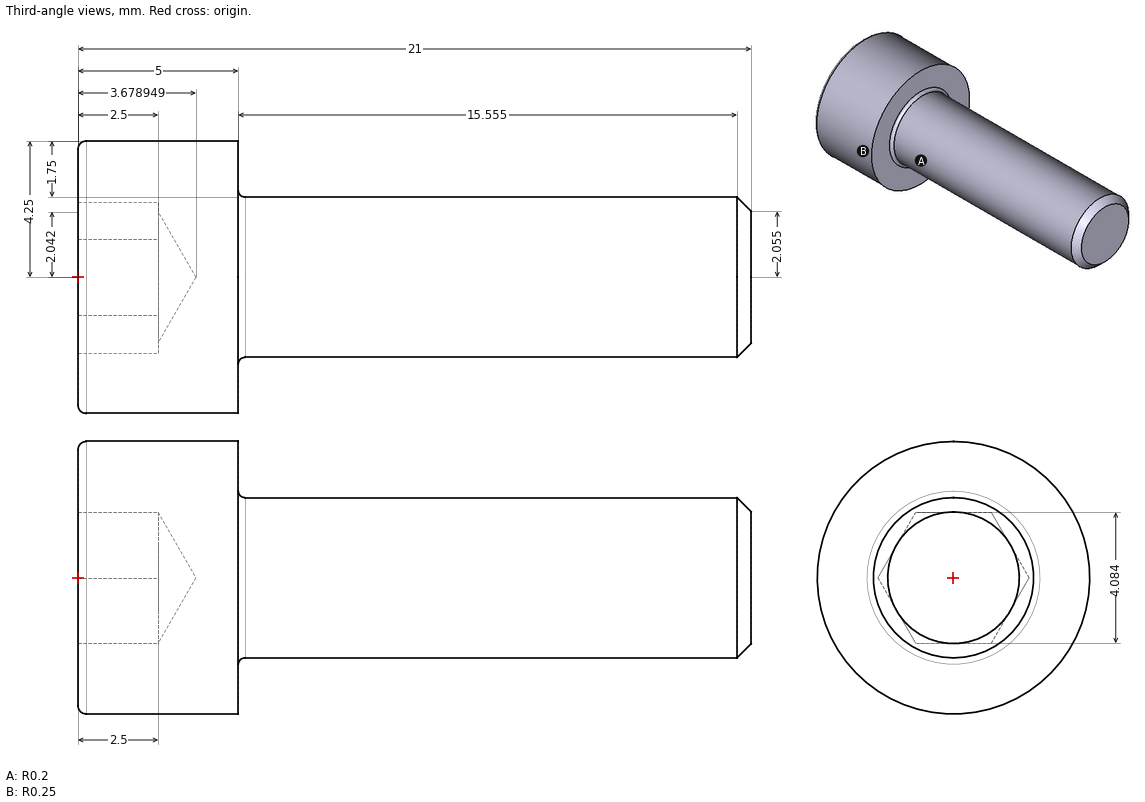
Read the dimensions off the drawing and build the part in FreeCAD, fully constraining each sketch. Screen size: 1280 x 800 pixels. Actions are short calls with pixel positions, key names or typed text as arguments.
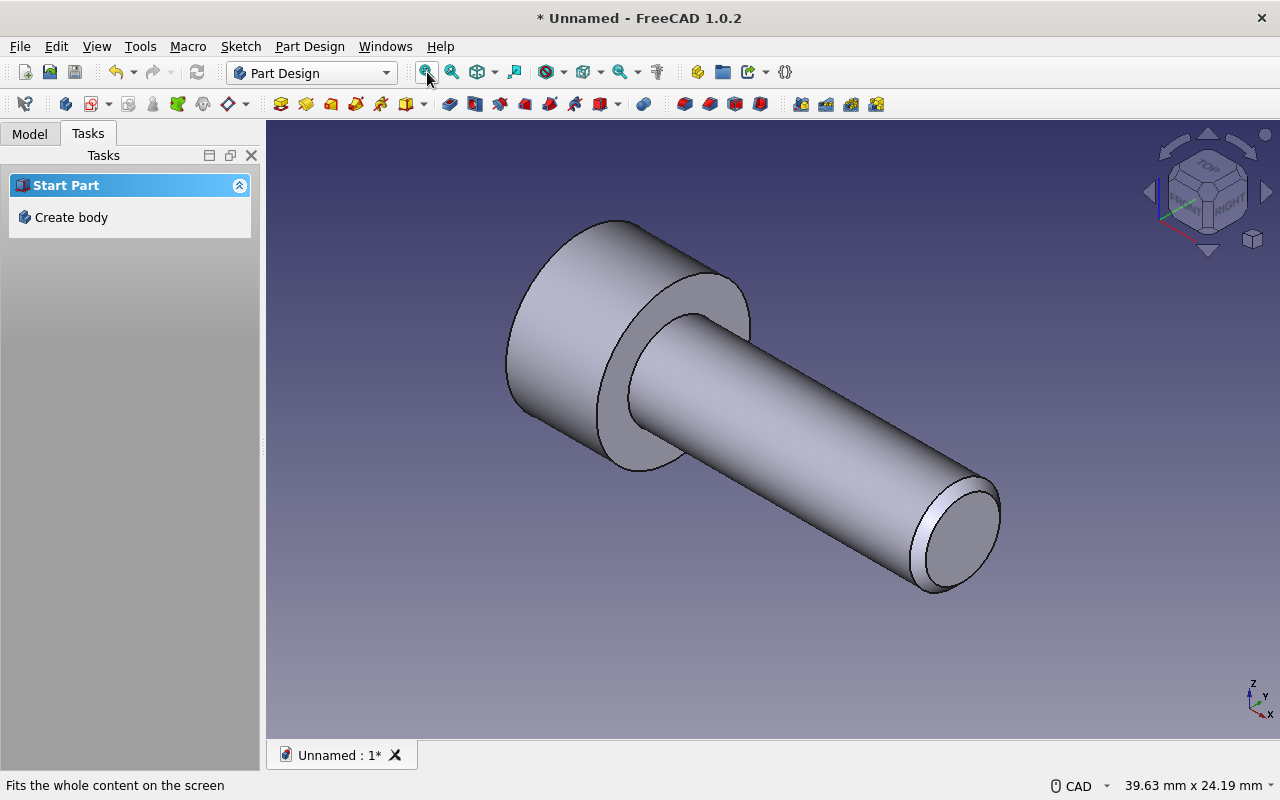
key(2)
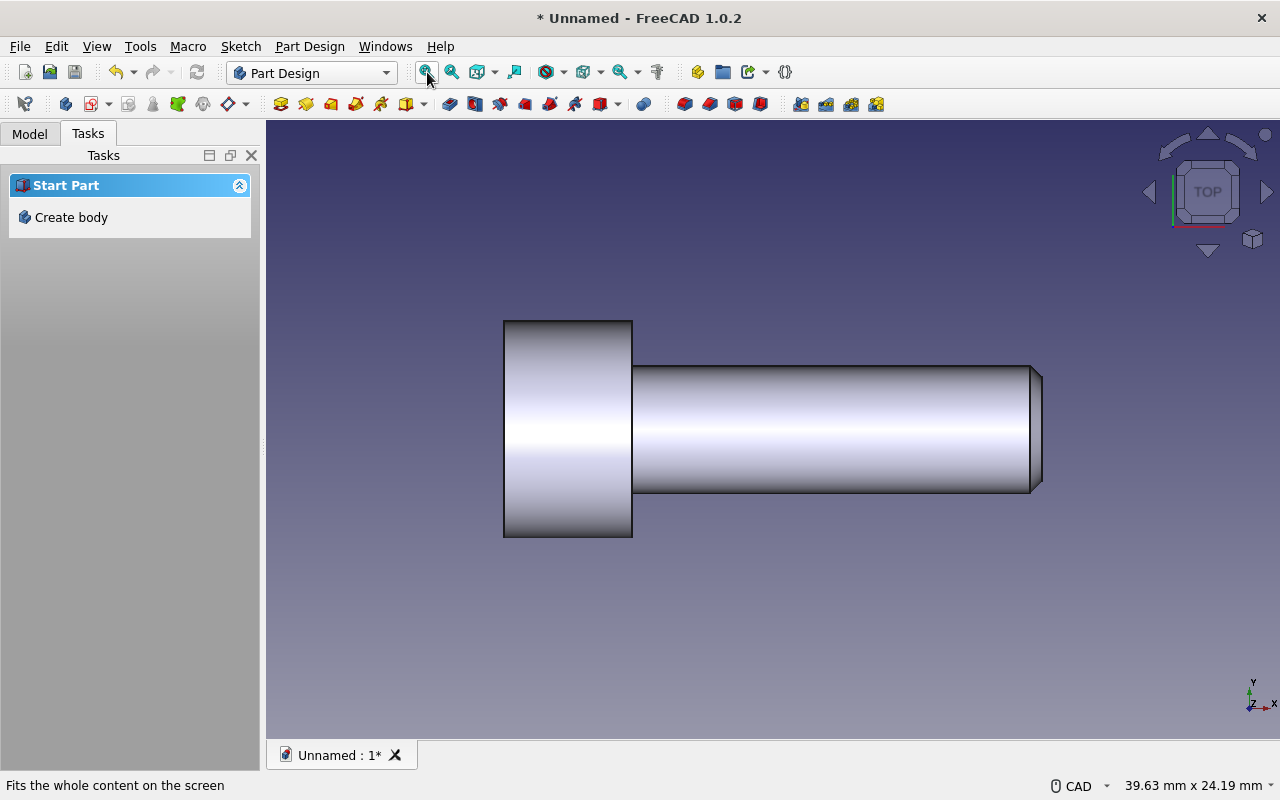
key(1)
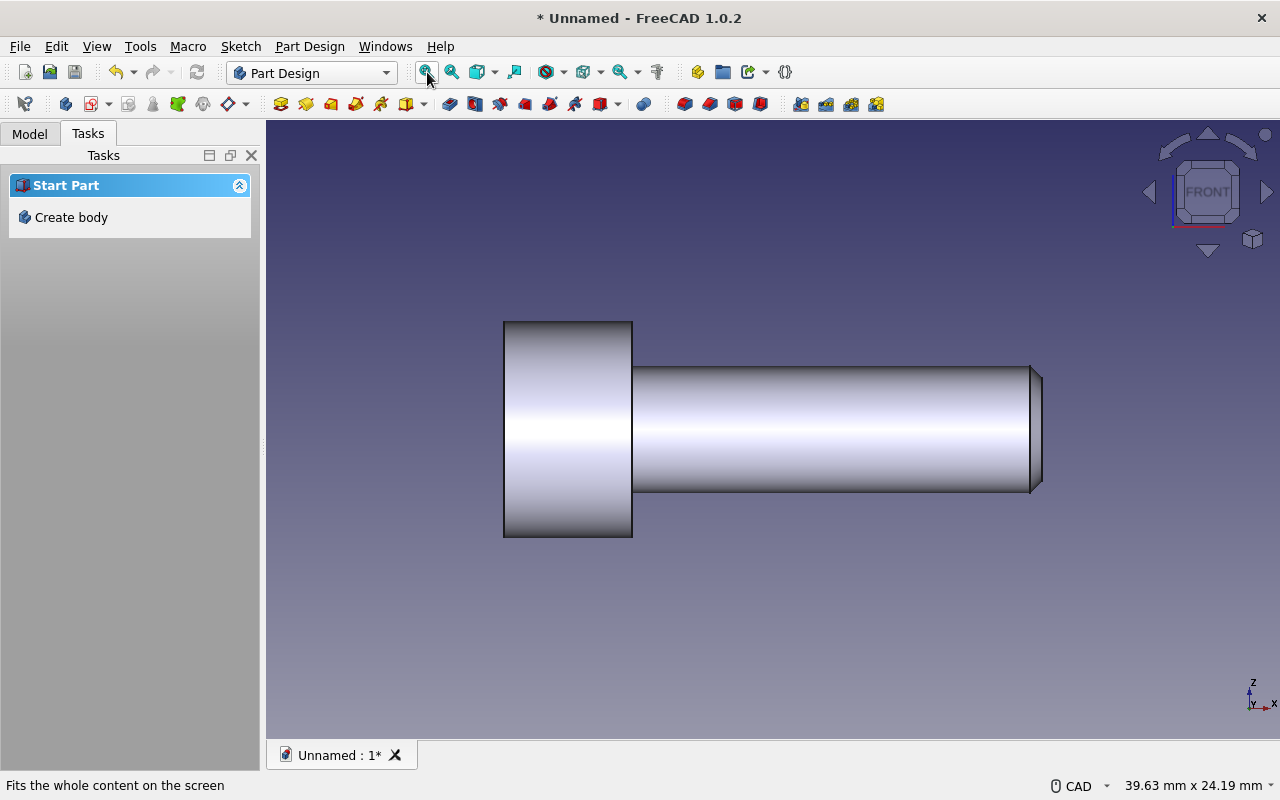
key(3)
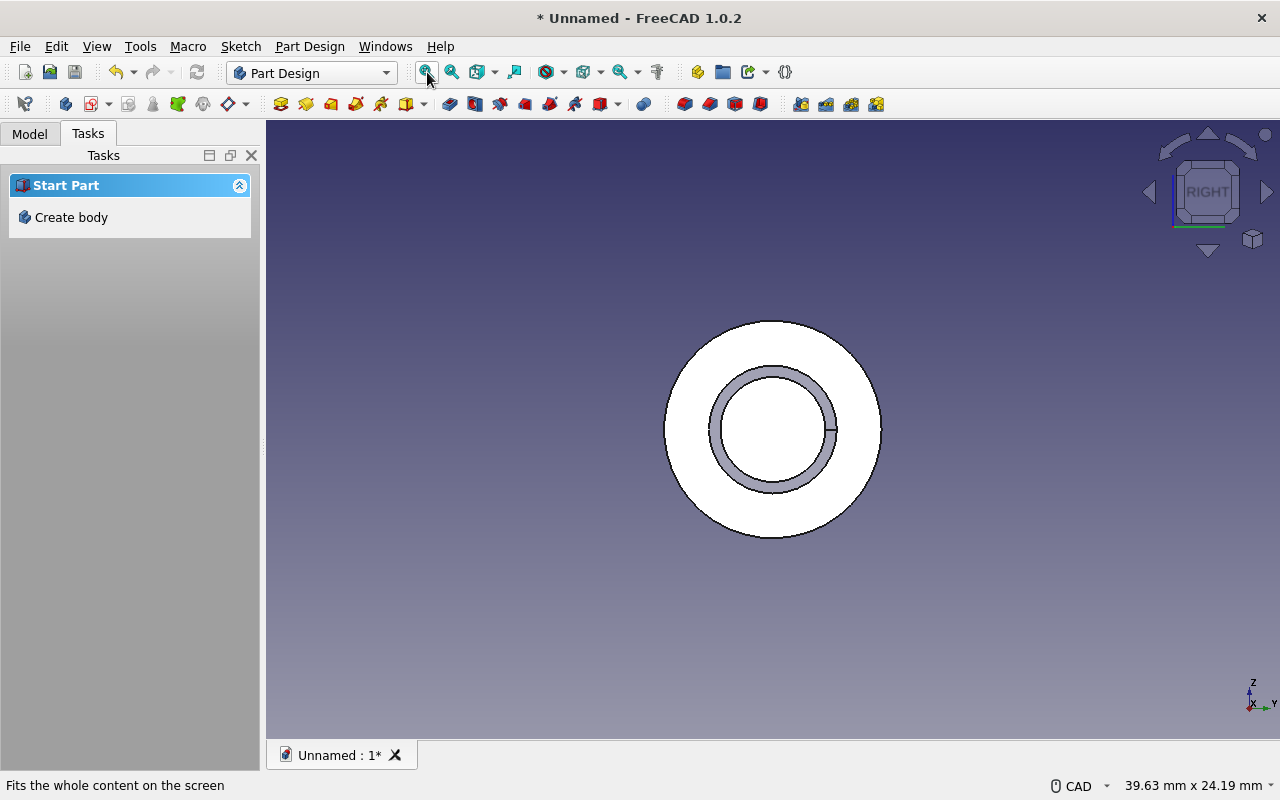
click(427, 72)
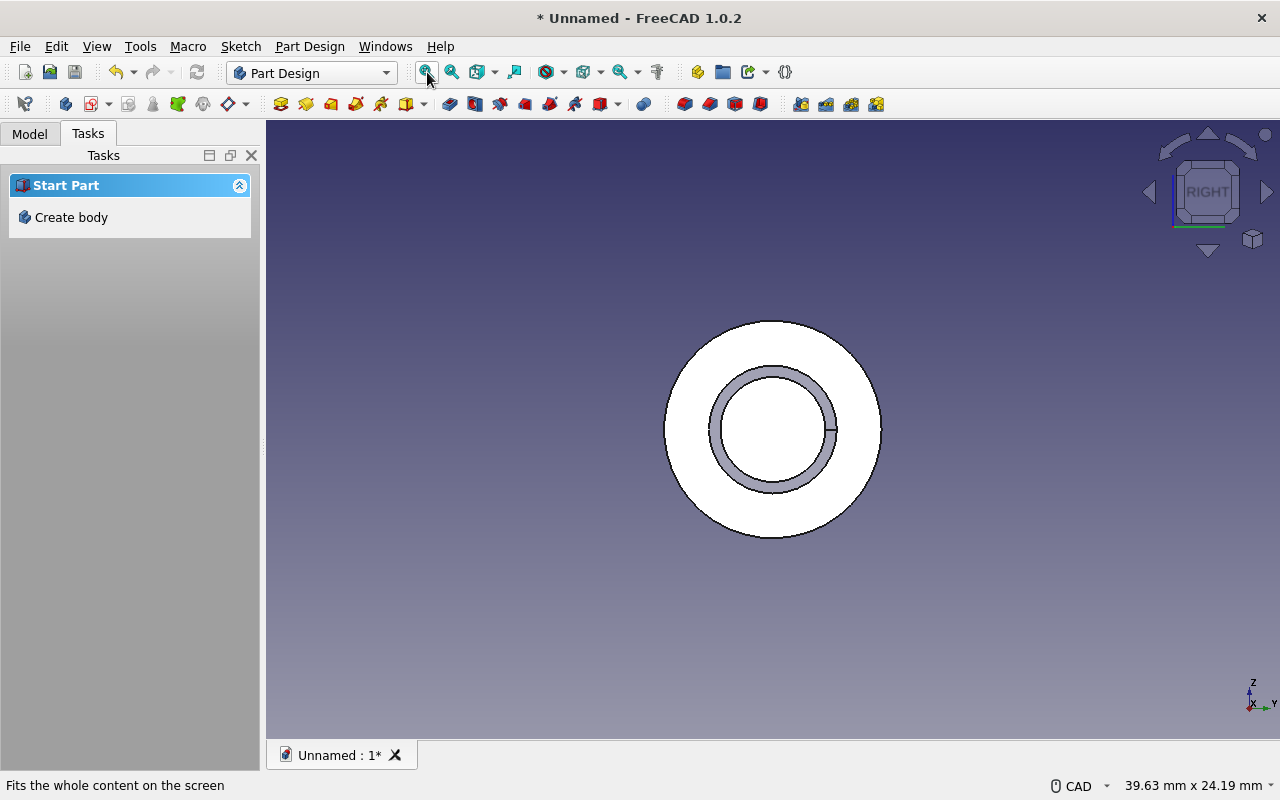
key(5)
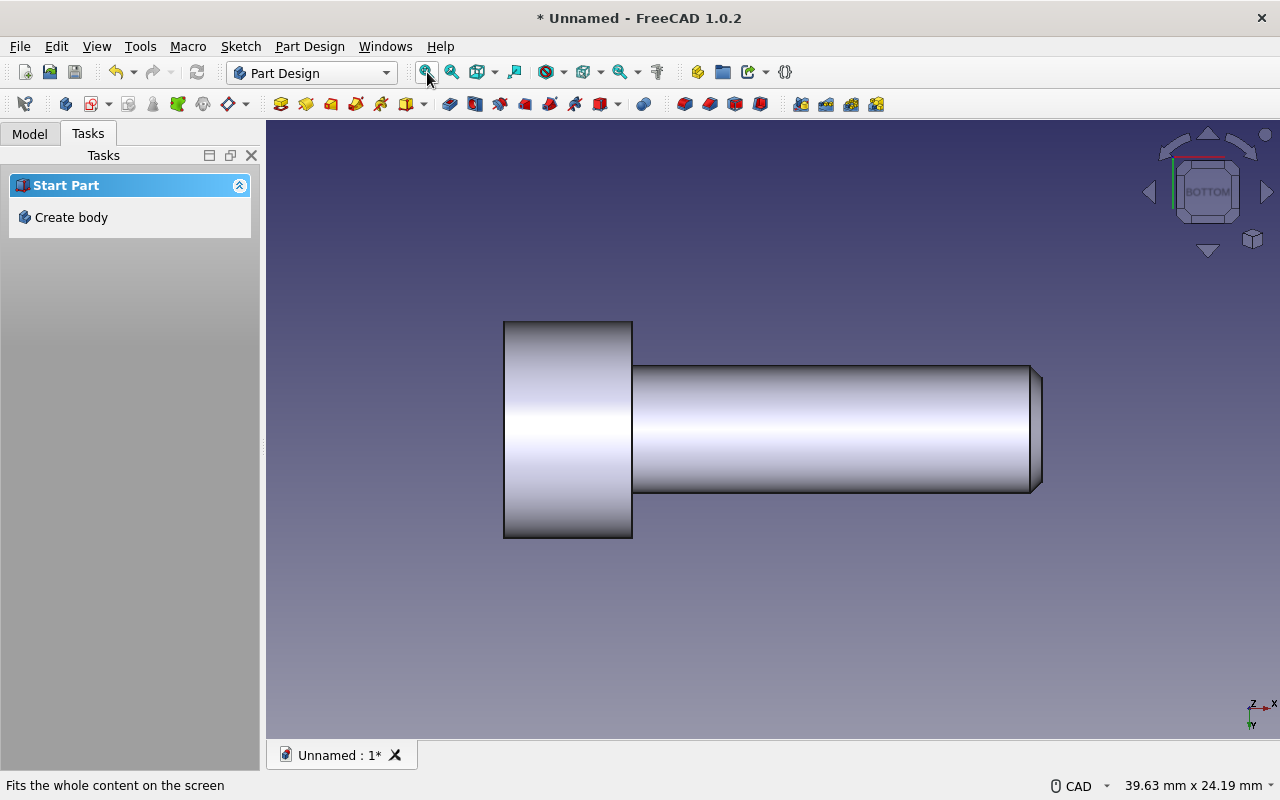
key(4)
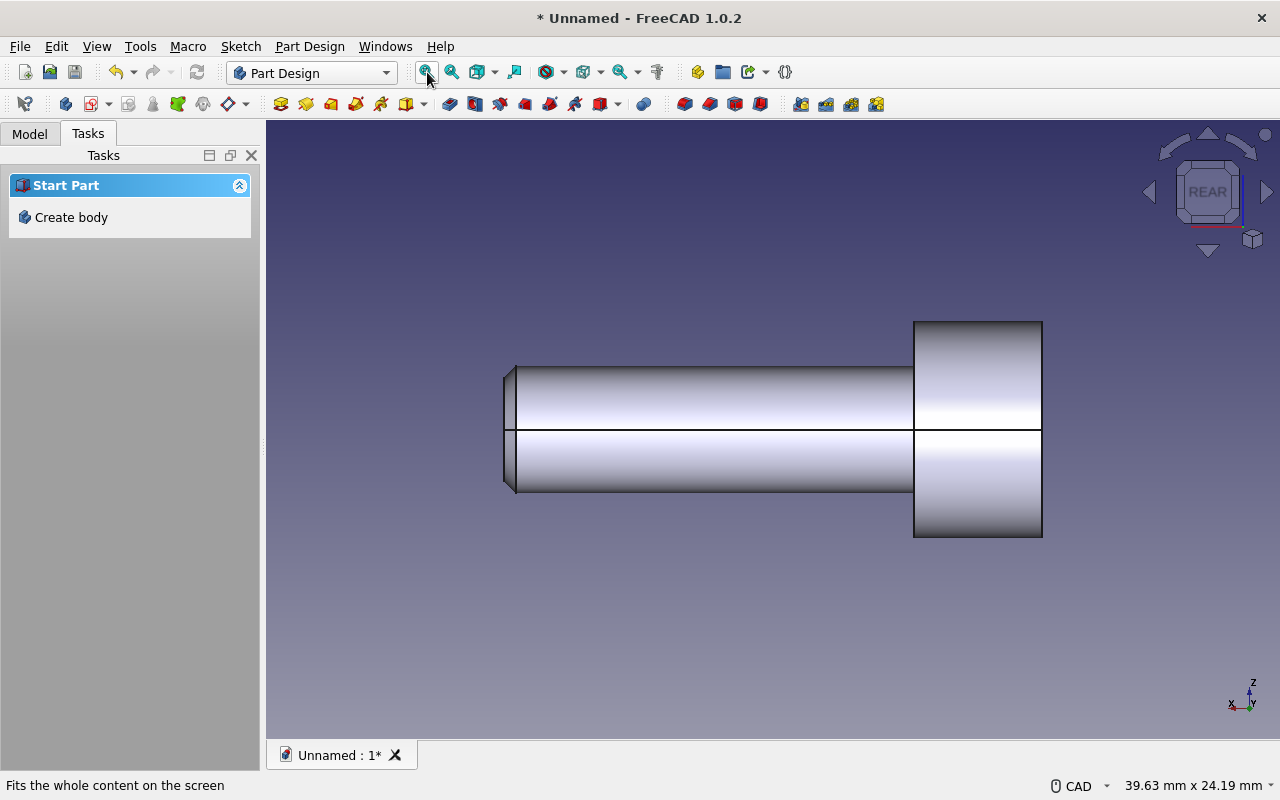
key(6)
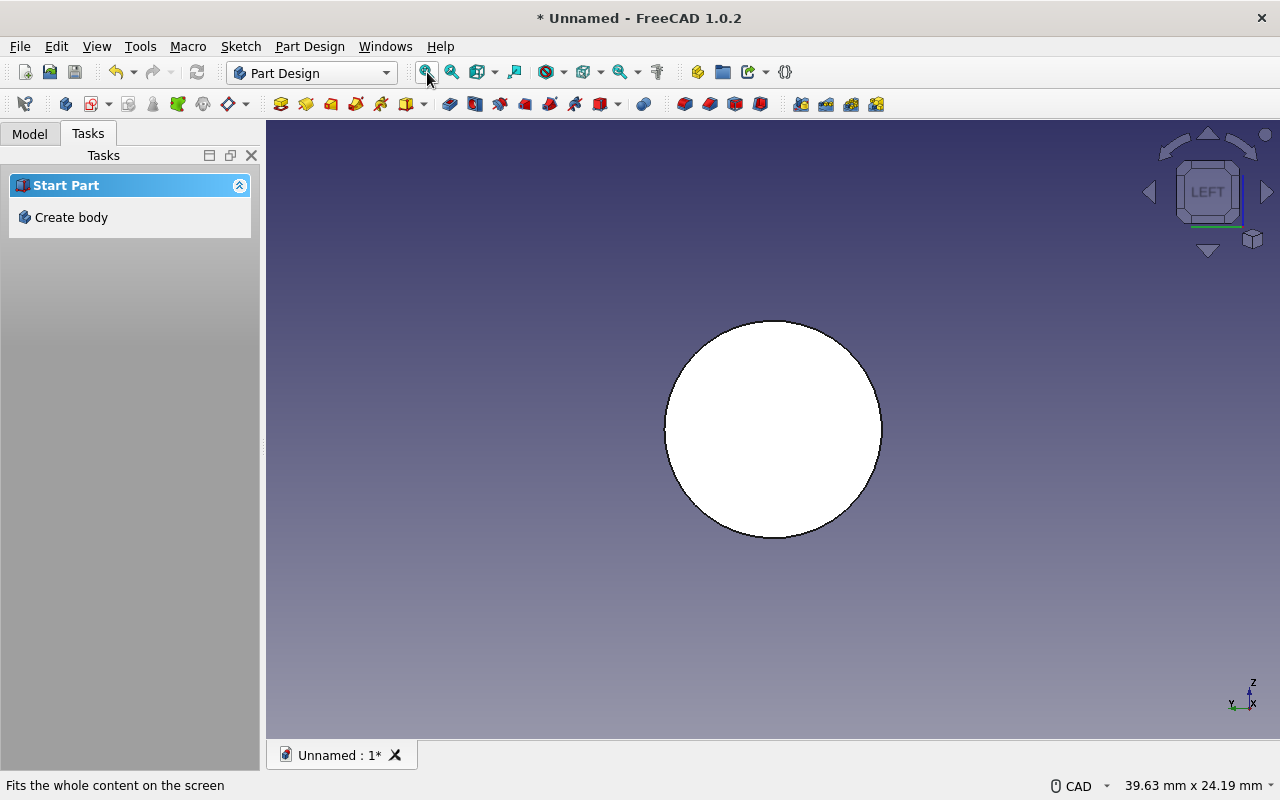
click(427, 72)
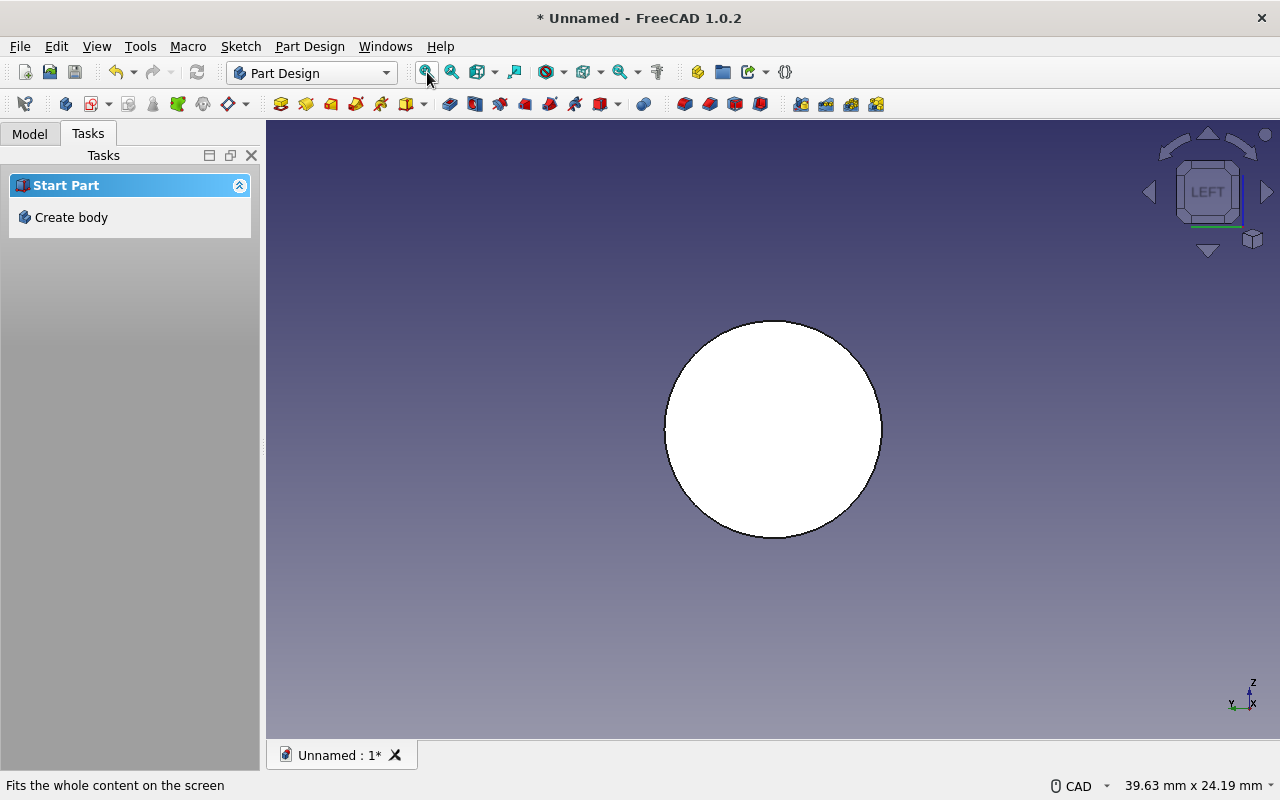
key(v)
key(3)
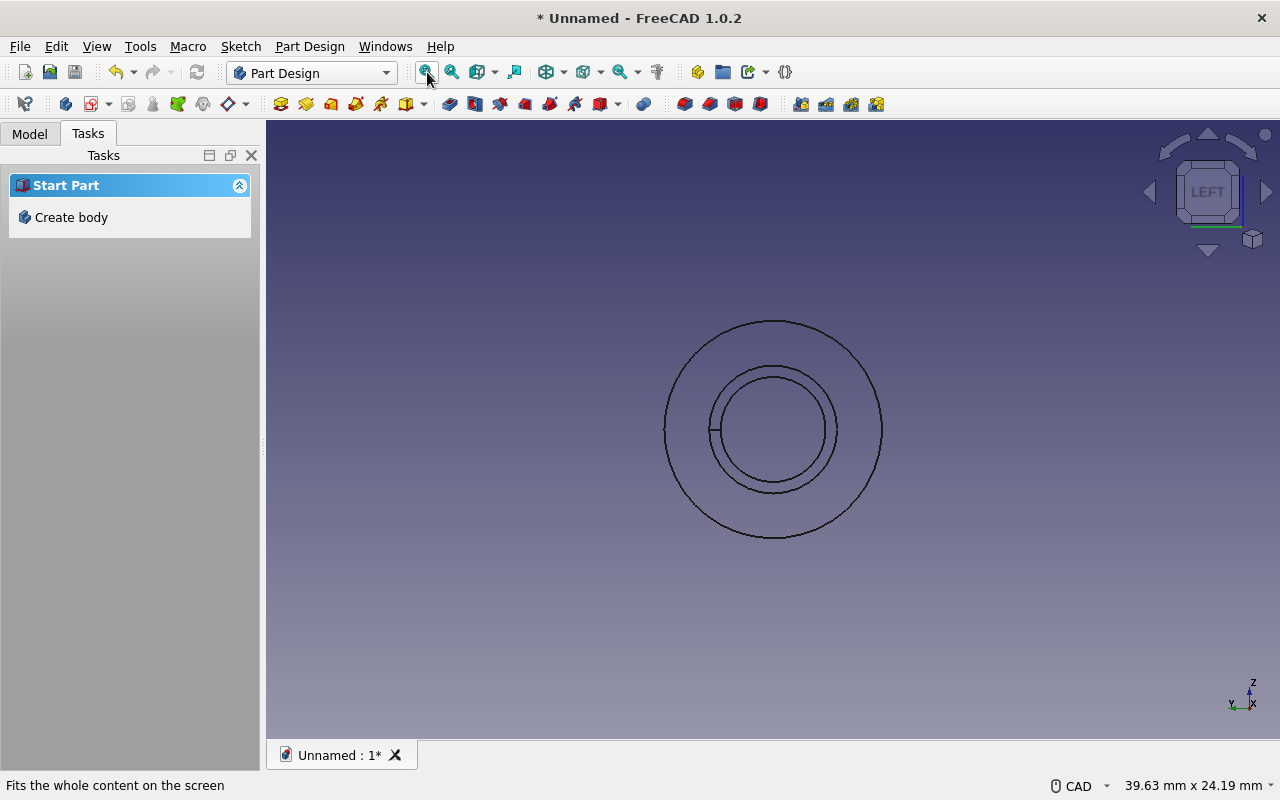
key(0)